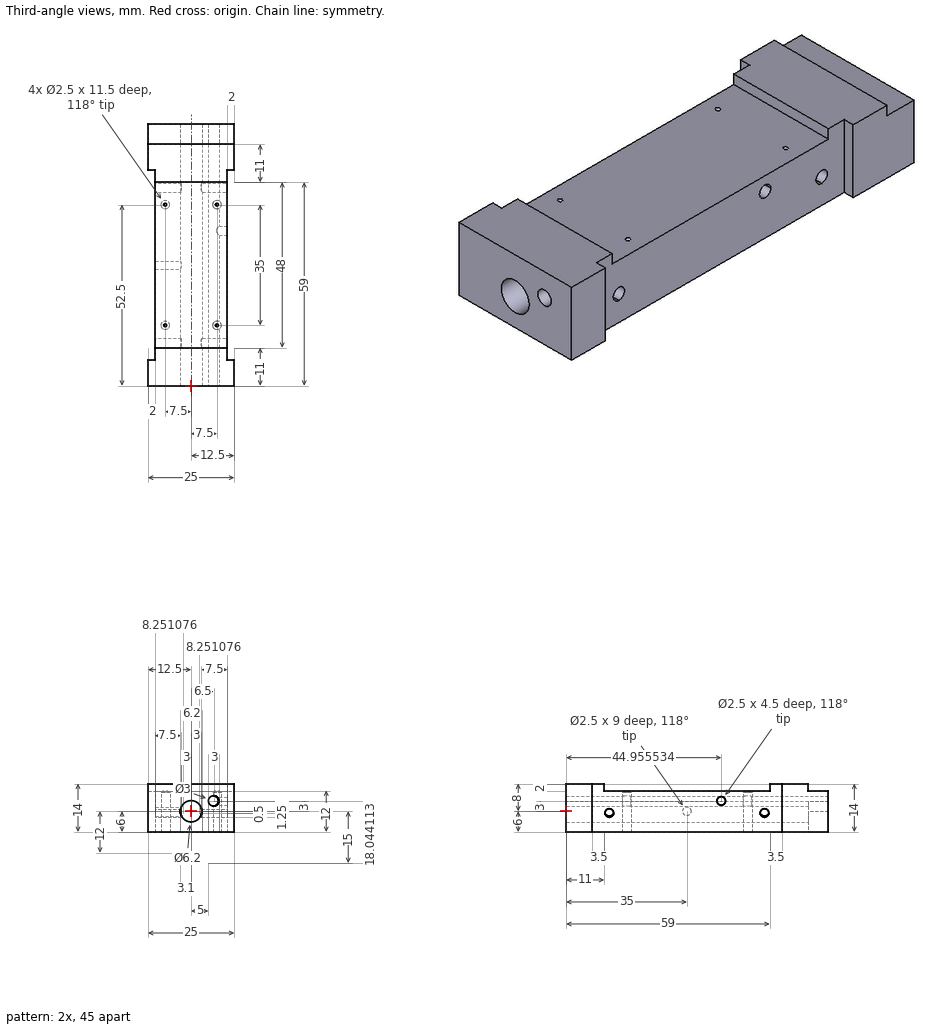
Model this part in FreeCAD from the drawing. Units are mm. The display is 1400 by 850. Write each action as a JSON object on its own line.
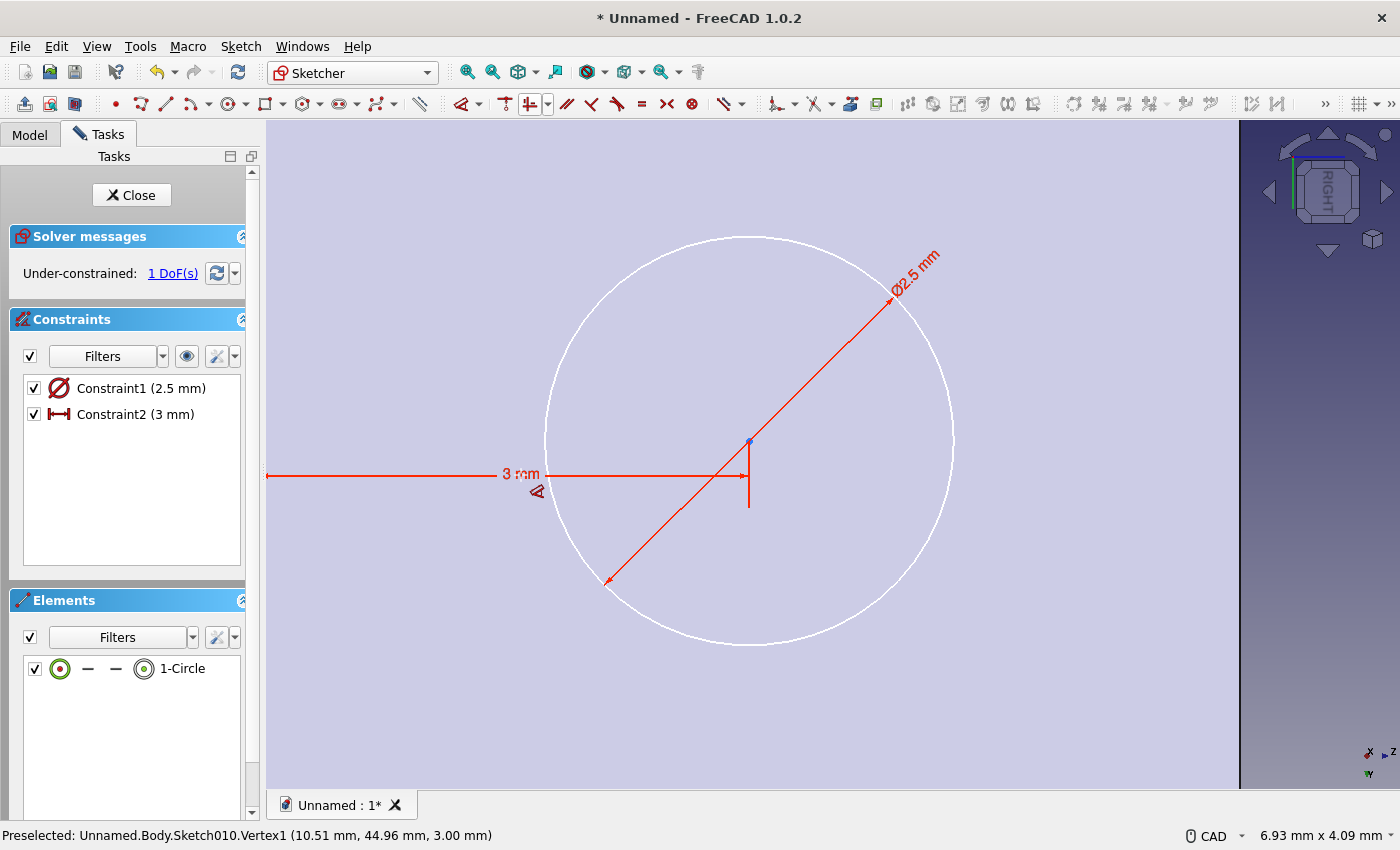
{"action": "left_click", "coordinate": [749, 441]}
{"action": "left_click", "coordinate": [783, 294]}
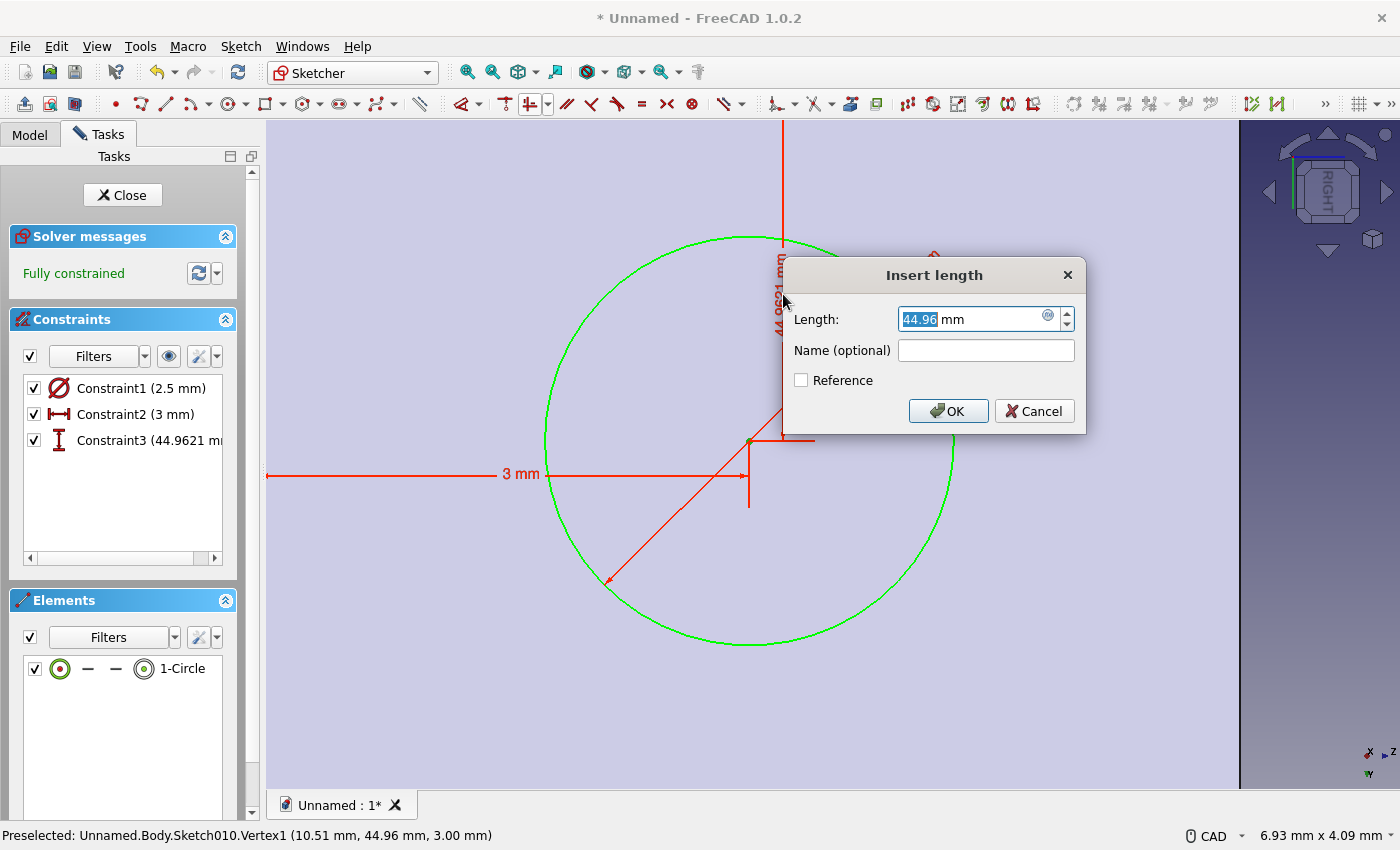
{"action": "type", "text": "44.955534"}
{"action": "key", "text": "Return"}
{"action": "key", "text": "Escape"}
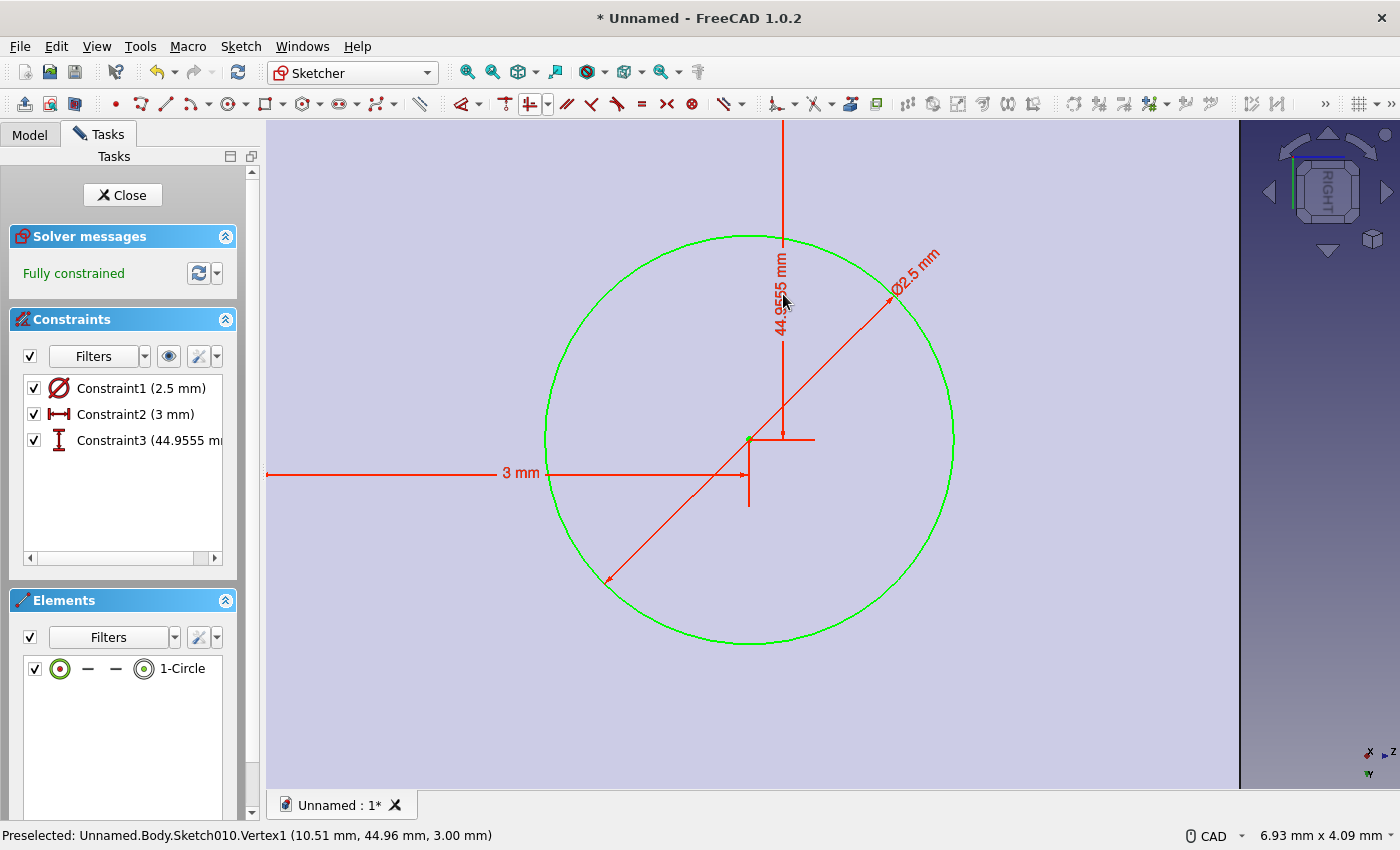
{"action": "left_click", "coordinate": [123, 195]}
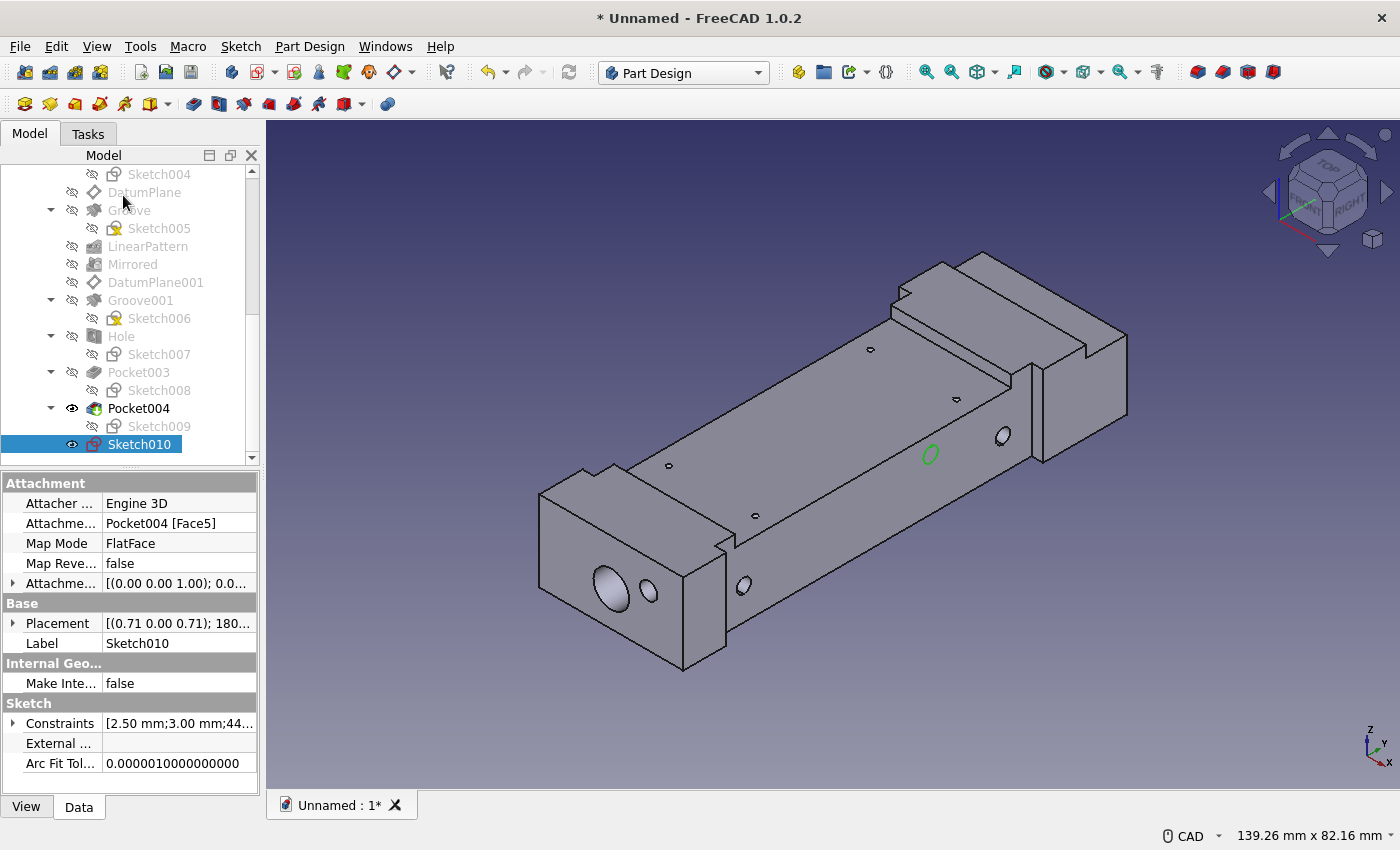
{"action": "left_click", "coordinate": [219, 104]}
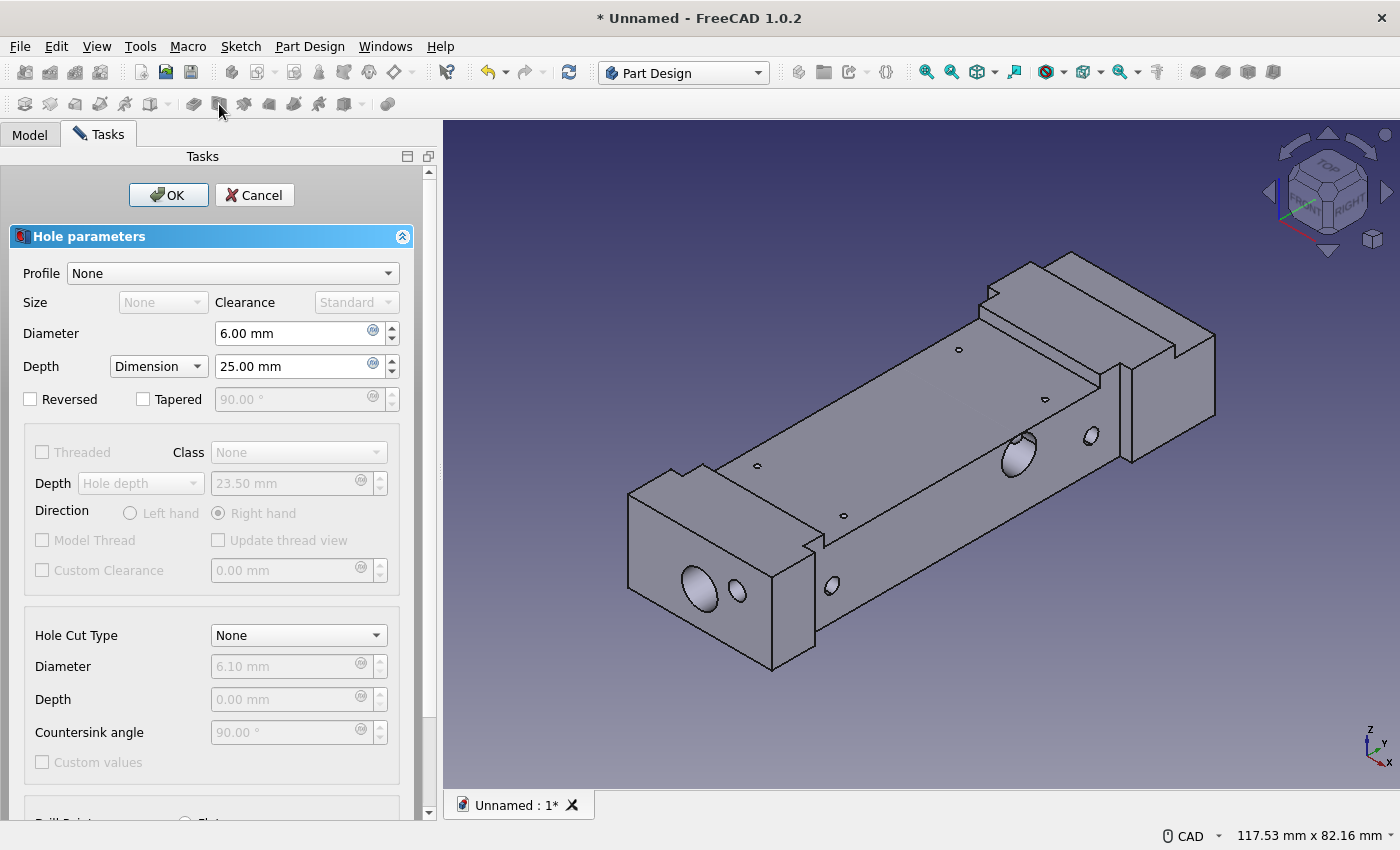
{"action": "triple_click", "coordinate": [300, 334]}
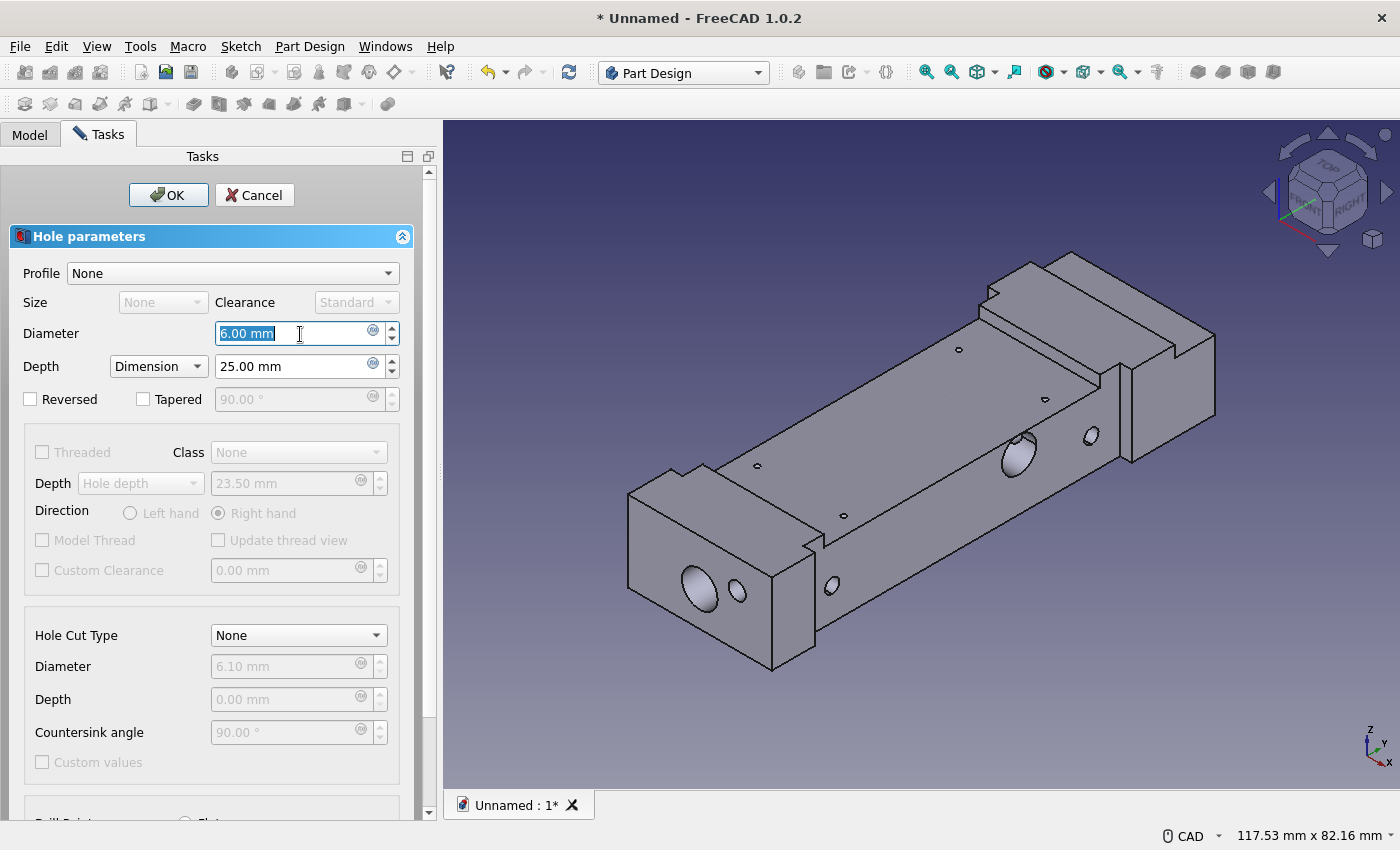
{"action": "type", "text": "2.5"}
{"action": "key", "text": "Tab"}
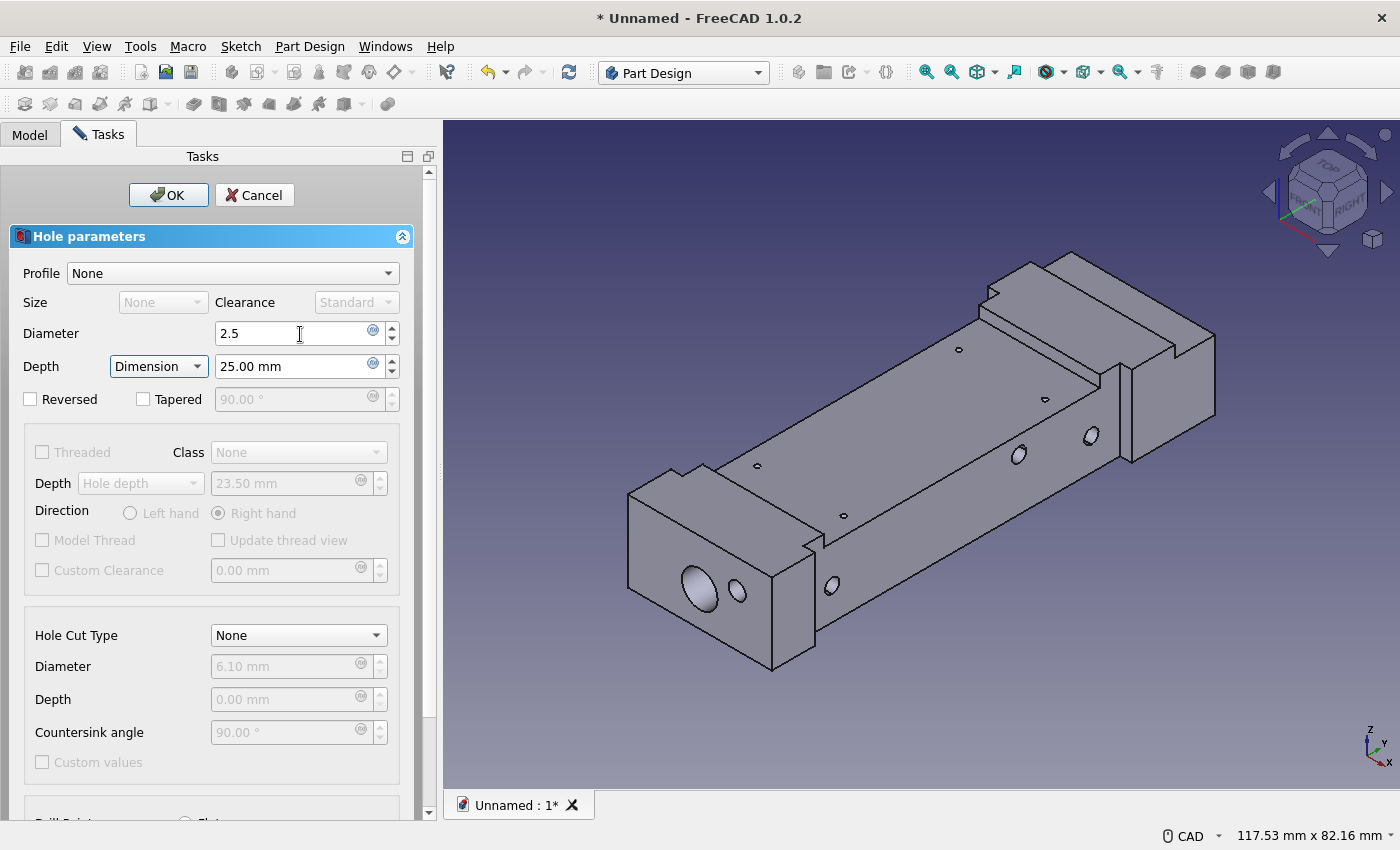
{"action": "triple_click", "coordinate": [300, 366]}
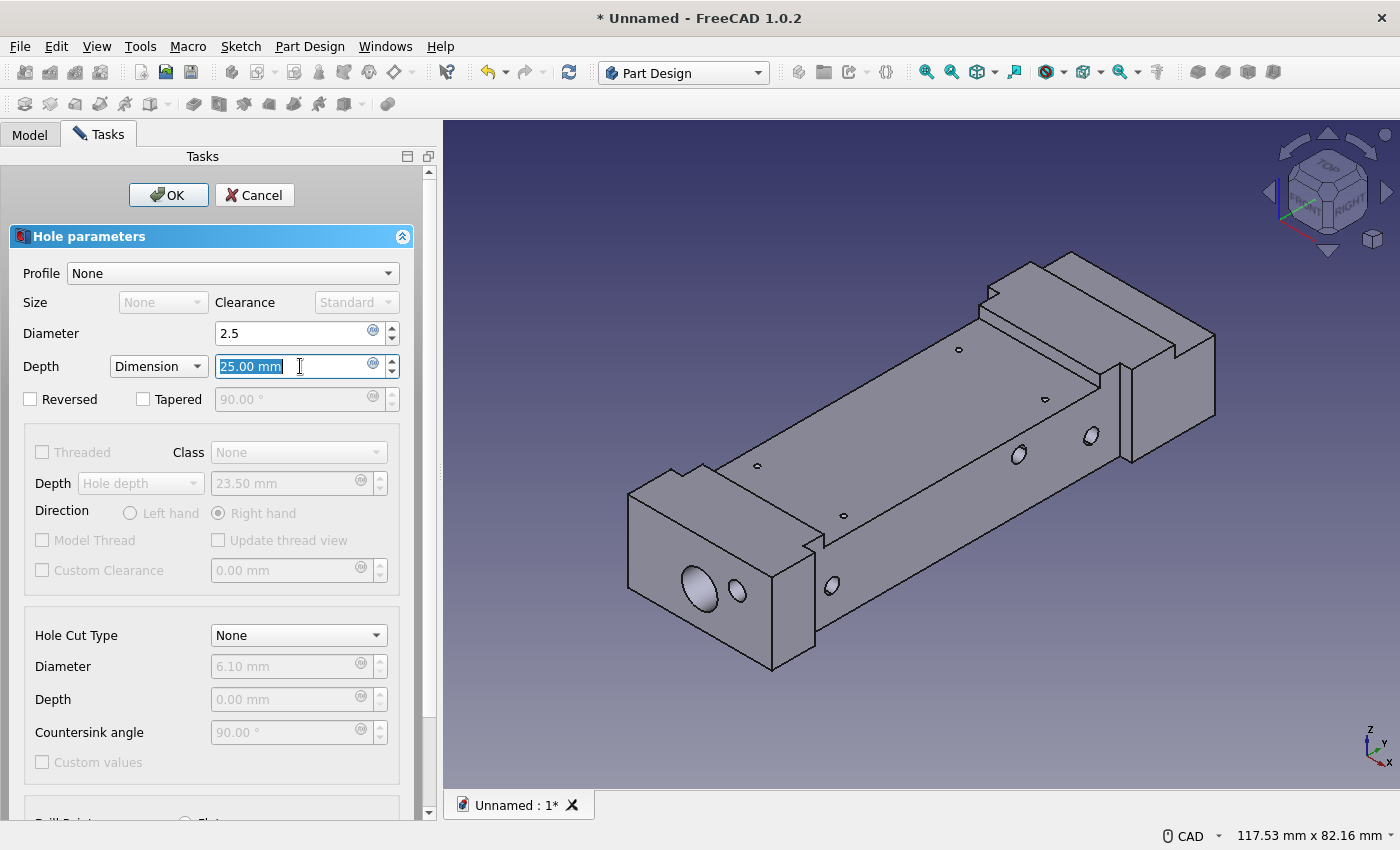
{"action": "type", "text": "4.5"}
{"action": "key", "text": "Tab"}